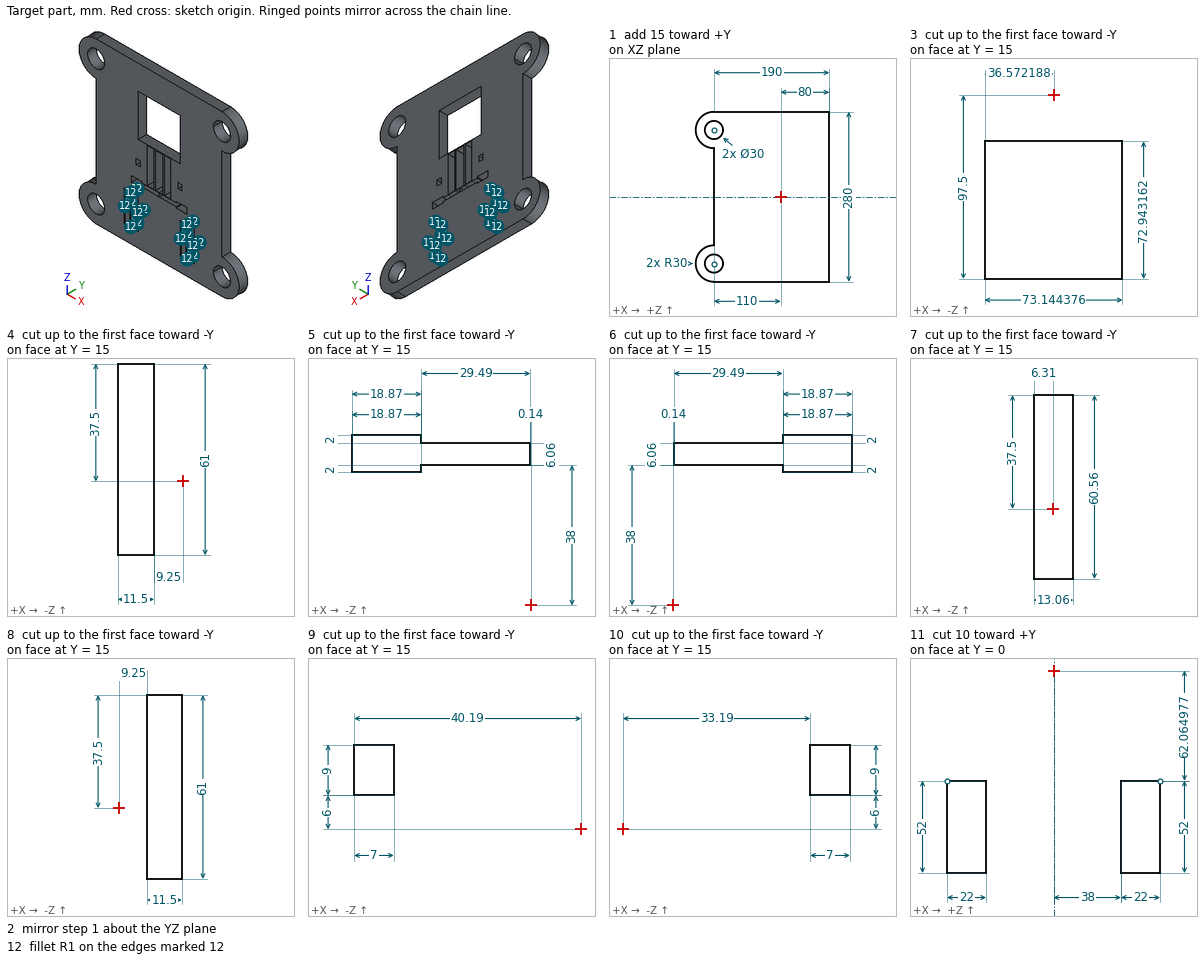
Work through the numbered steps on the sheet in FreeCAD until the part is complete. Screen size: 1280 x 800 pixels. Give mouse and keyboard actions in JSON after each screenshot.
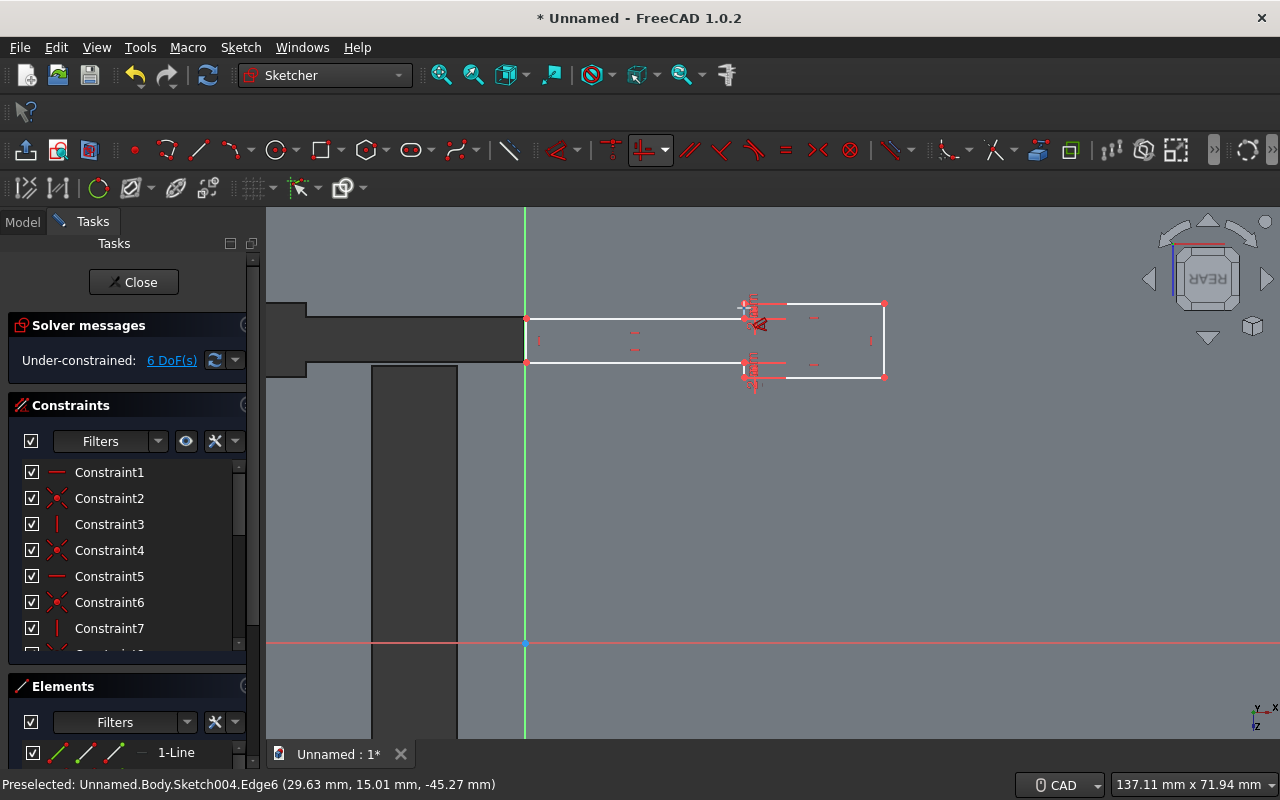
{"action": "left_click", "coordinate": [526, 363]}
{"action": "left_click", "coordinate": [491, 503]}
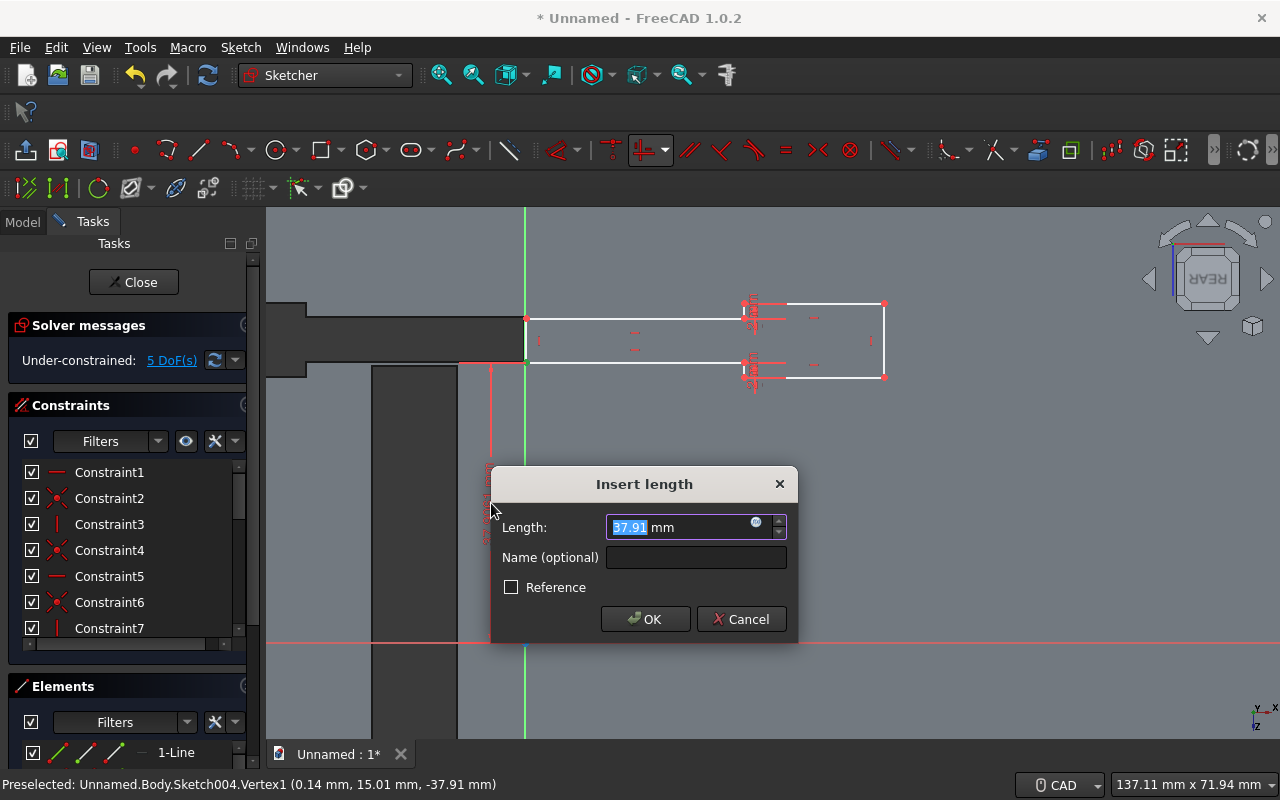
{"action": "type", "text": "38"}
{"action": "key", "text": "Return"}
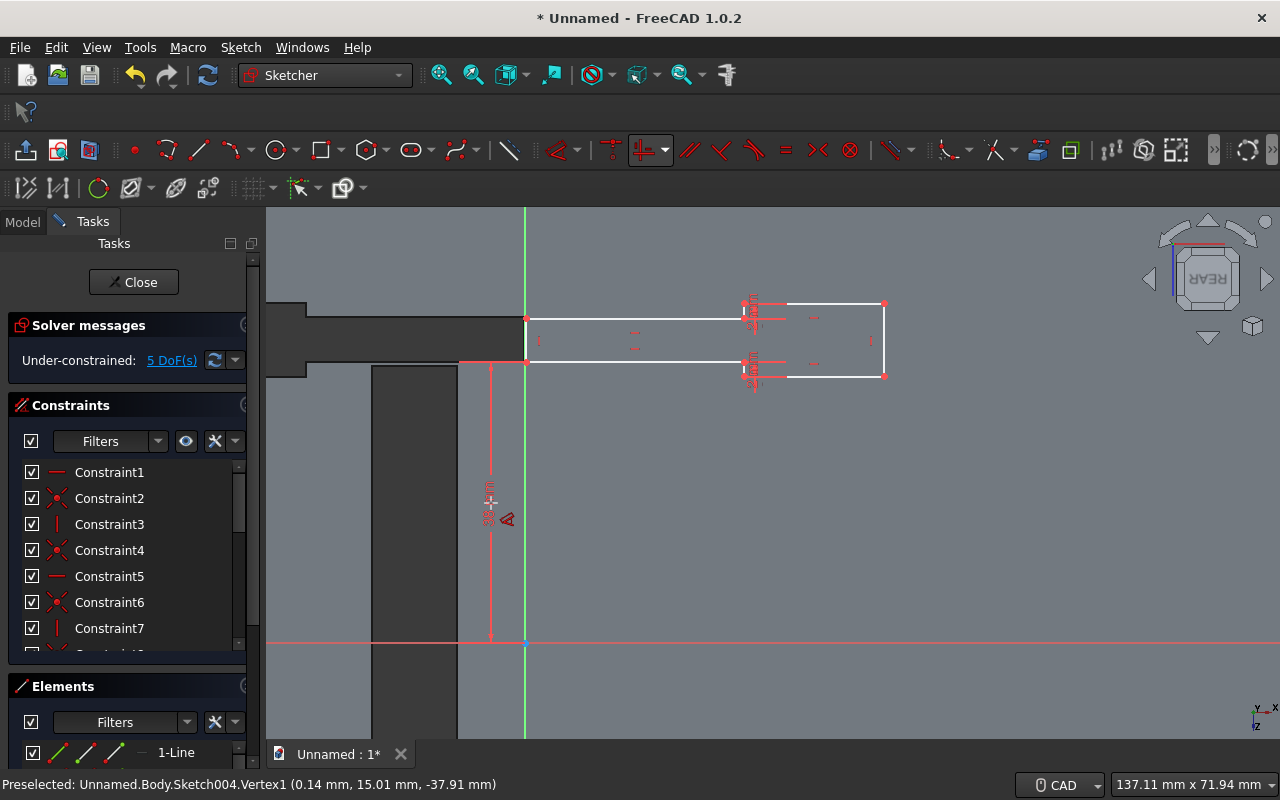
{"action": "left_click", "coordinate": [526, 332]}
{"action": "left_click", "coordinate": [492, 340]}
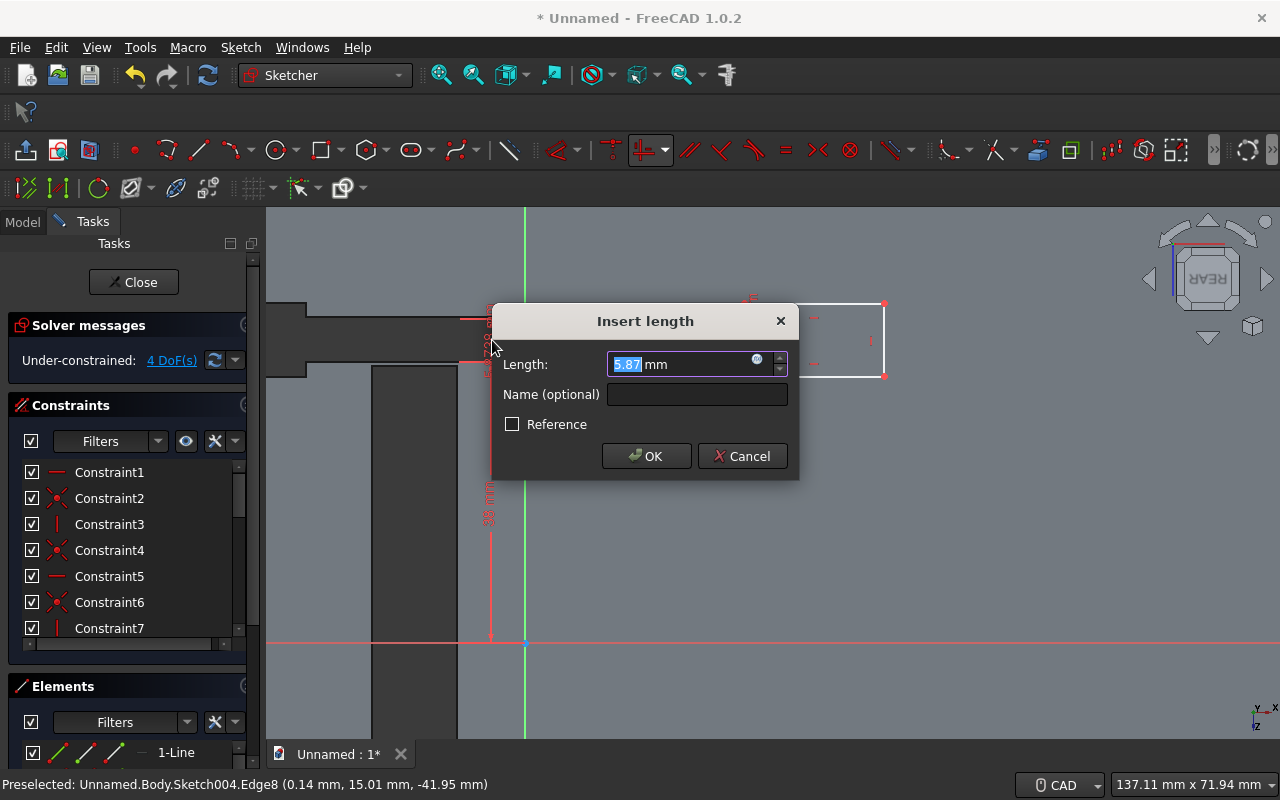
{"action": "type", "text": "6.06"}
{"action": "key", "text": "Return"}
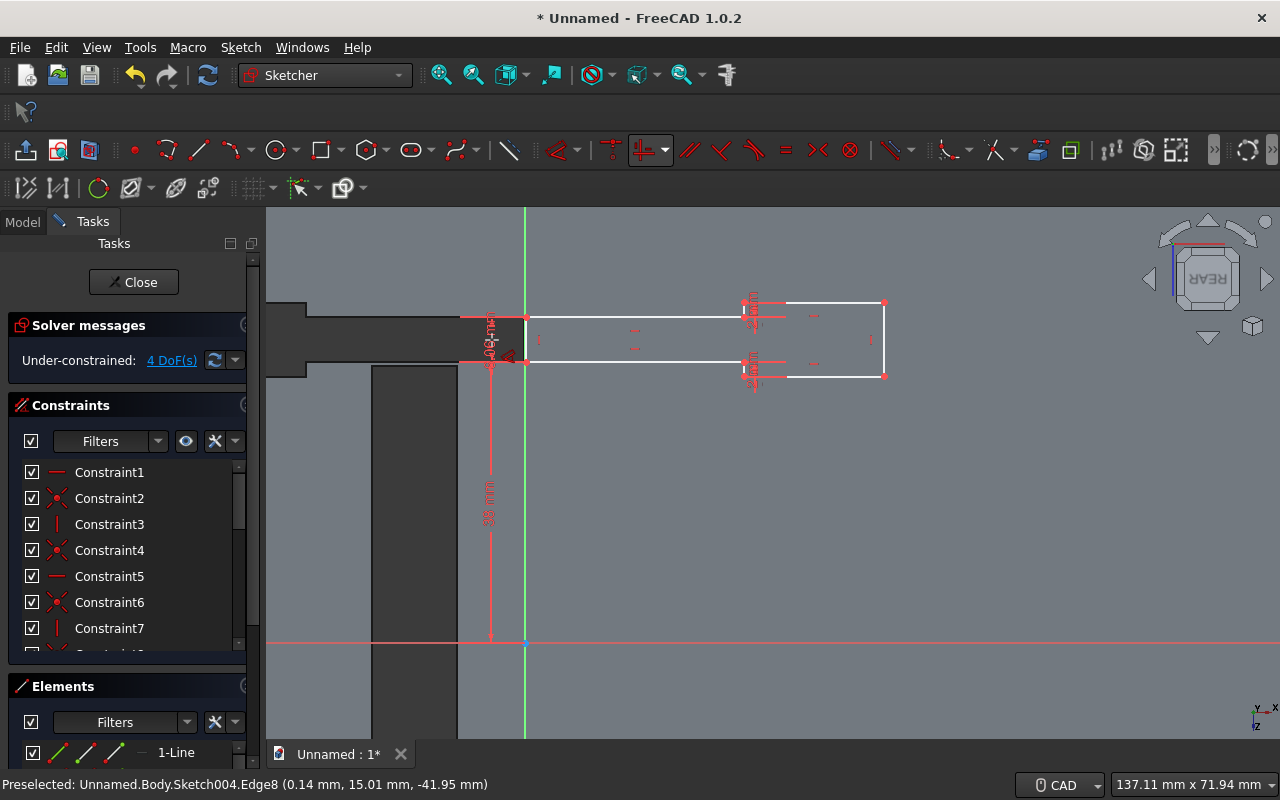
{"action": "left_click", "coordinate": [592, 362]}
{"action": "left_click", "coordinate": [635, 396]}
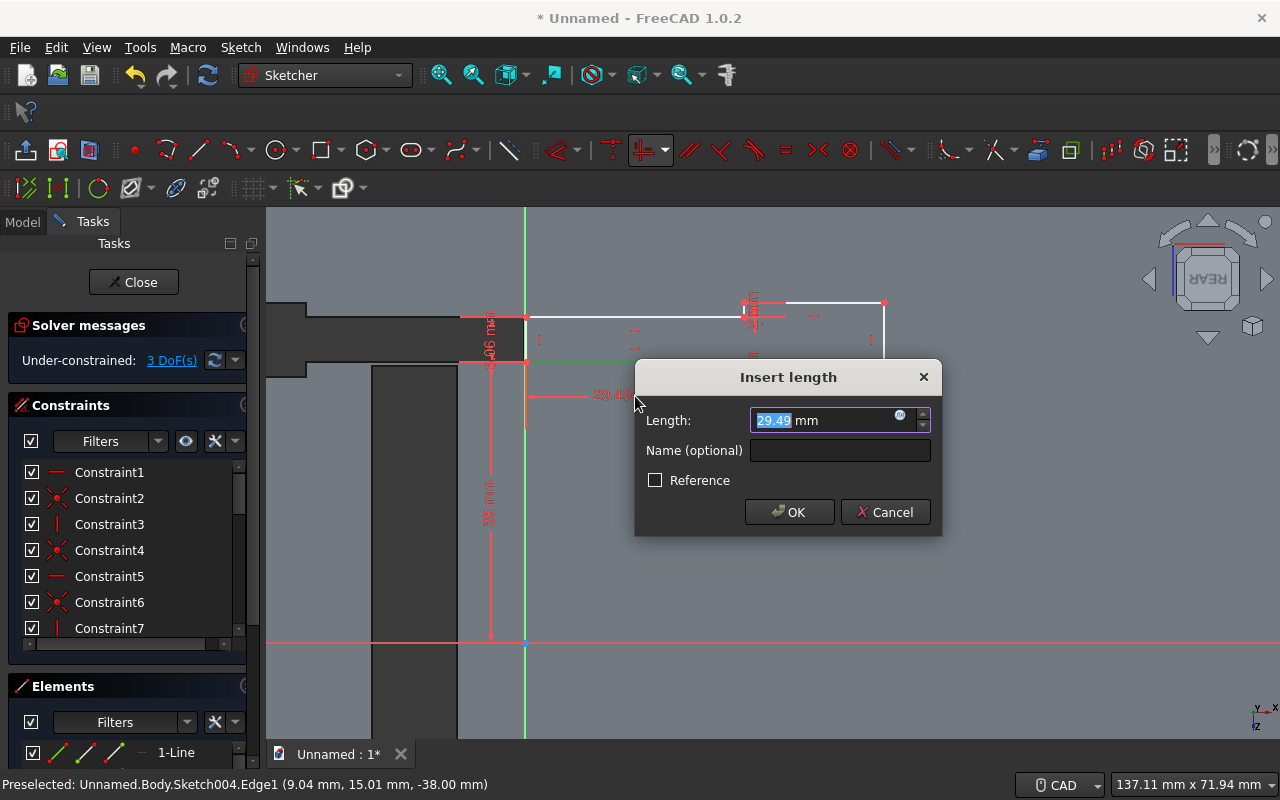
{"action": "type", "text": "29.49"}
{"action": "key", "text": "Return"}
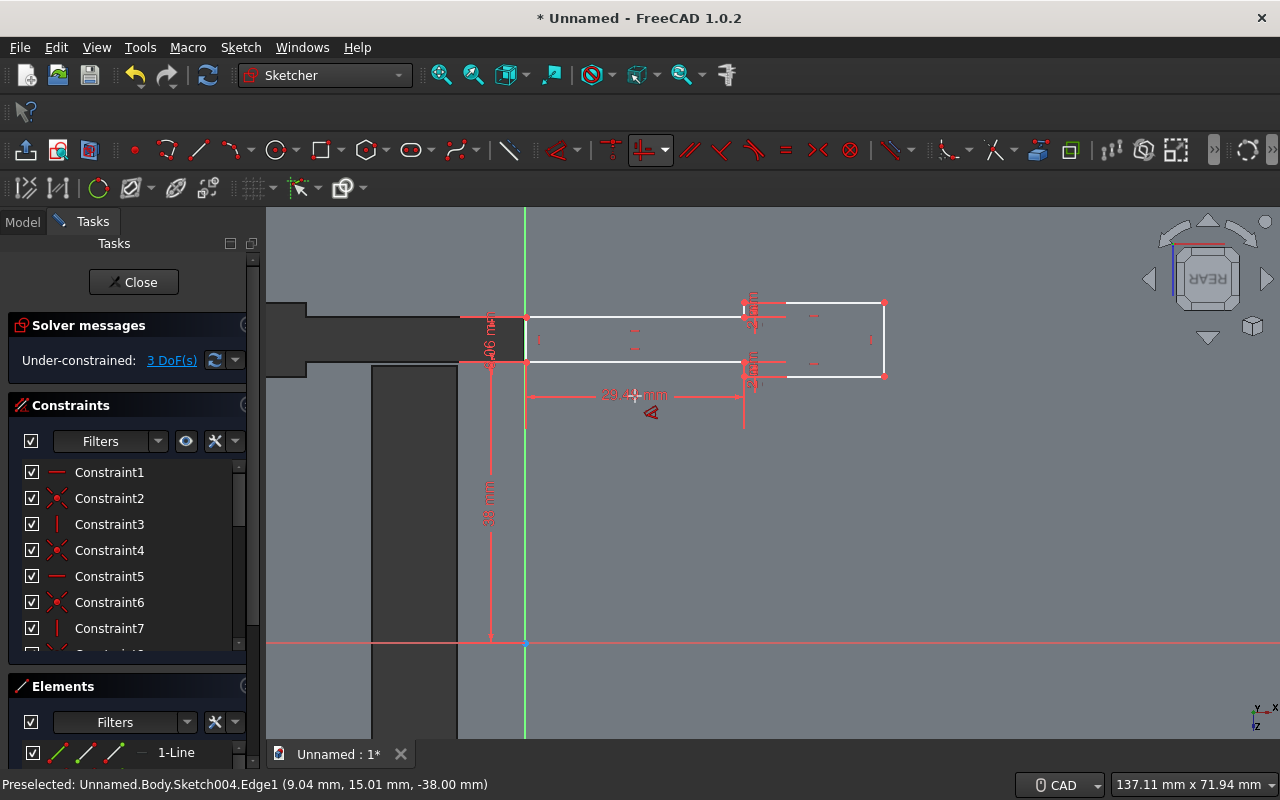
{"action": "left_click", "coordinate": [786, 377]}
{"action": "left_click", "coordinate": [814, 343]}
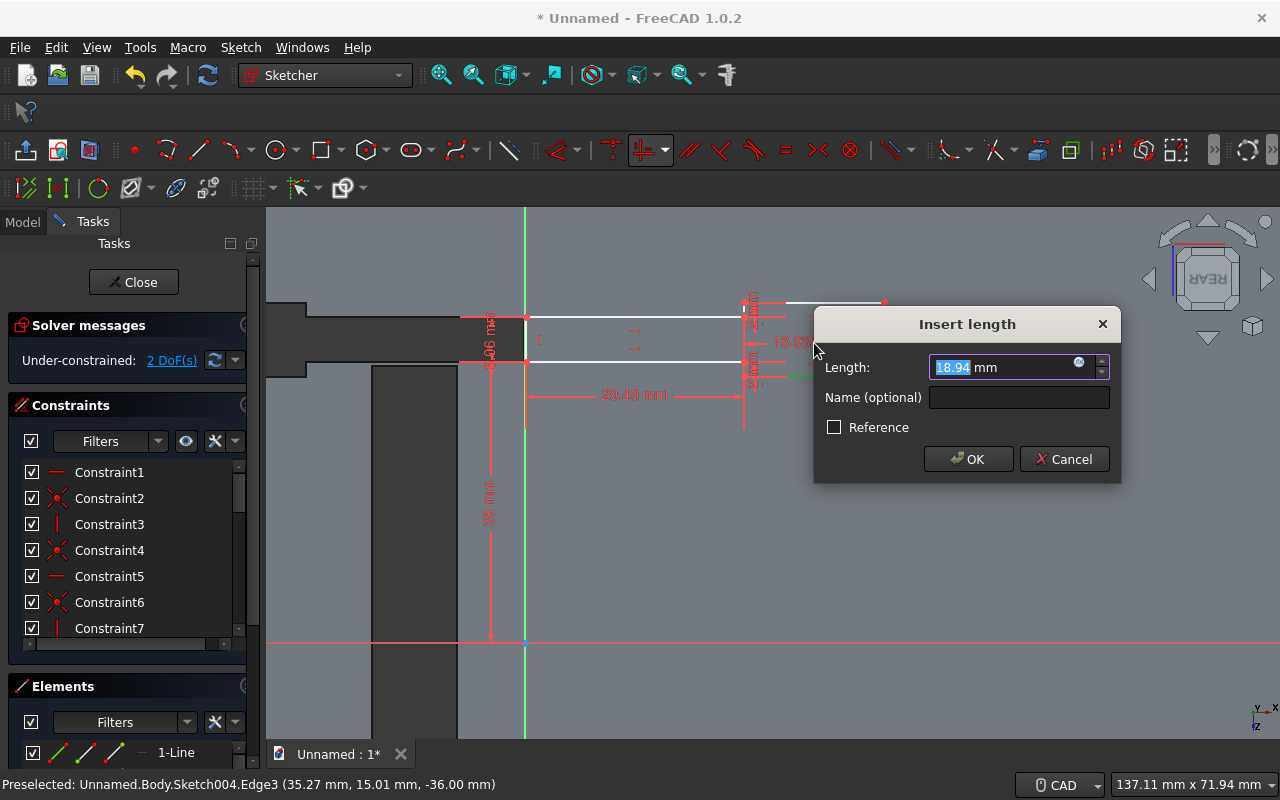
{"action": "type", "text": "18.87"}
{"action": "key", "text": "Return"}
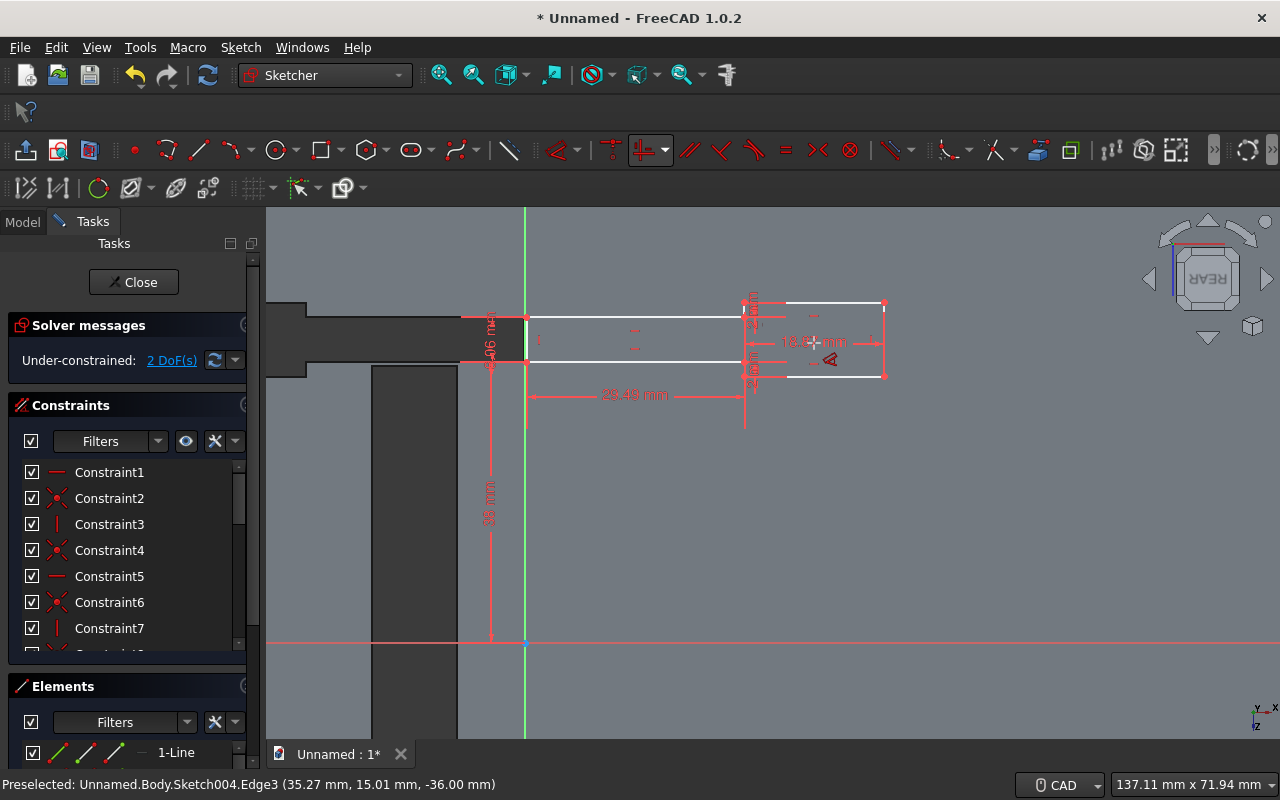
{"action": "left_click", "coordinate": [842, 303]}
{"action": "left_click", "coordinate": [814, 269]}